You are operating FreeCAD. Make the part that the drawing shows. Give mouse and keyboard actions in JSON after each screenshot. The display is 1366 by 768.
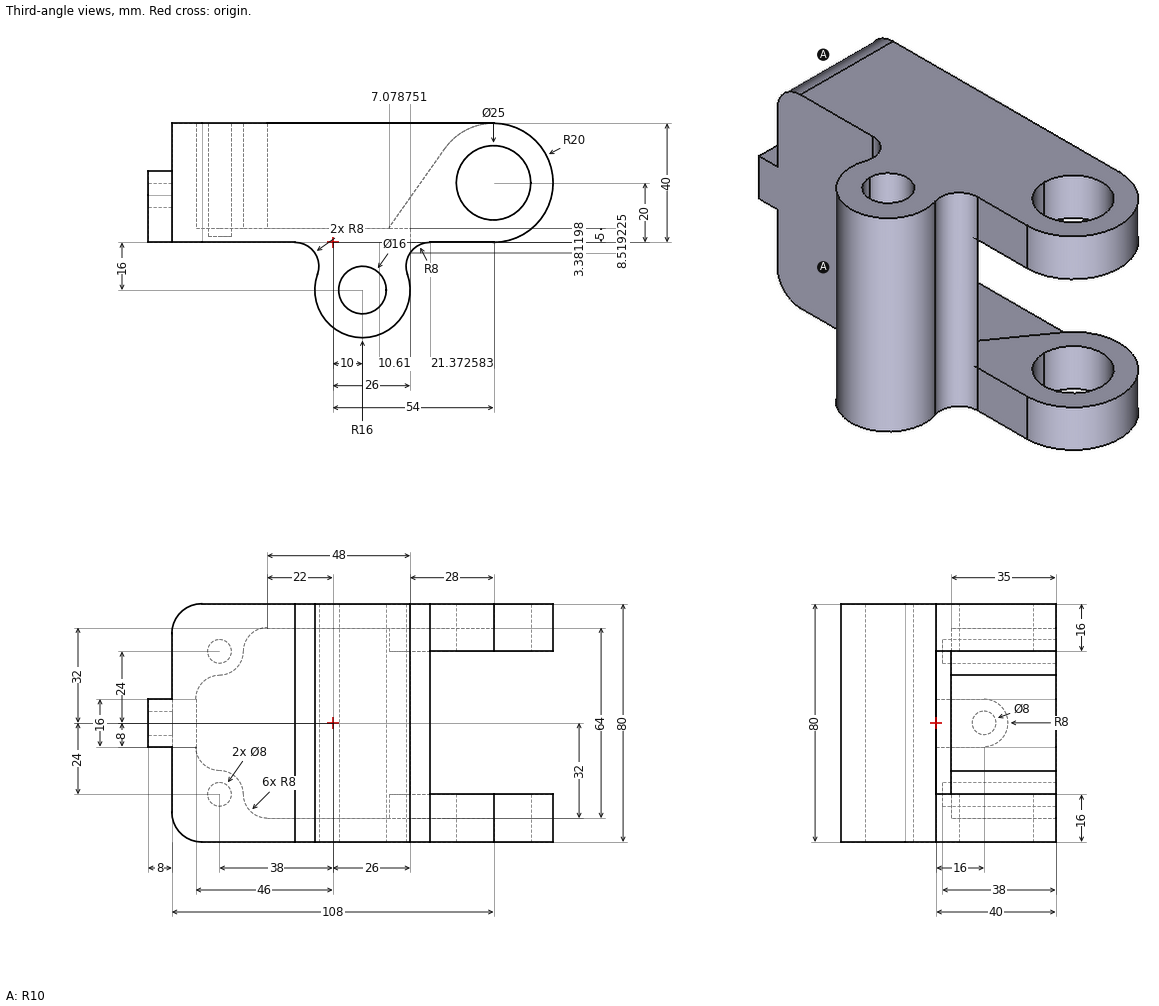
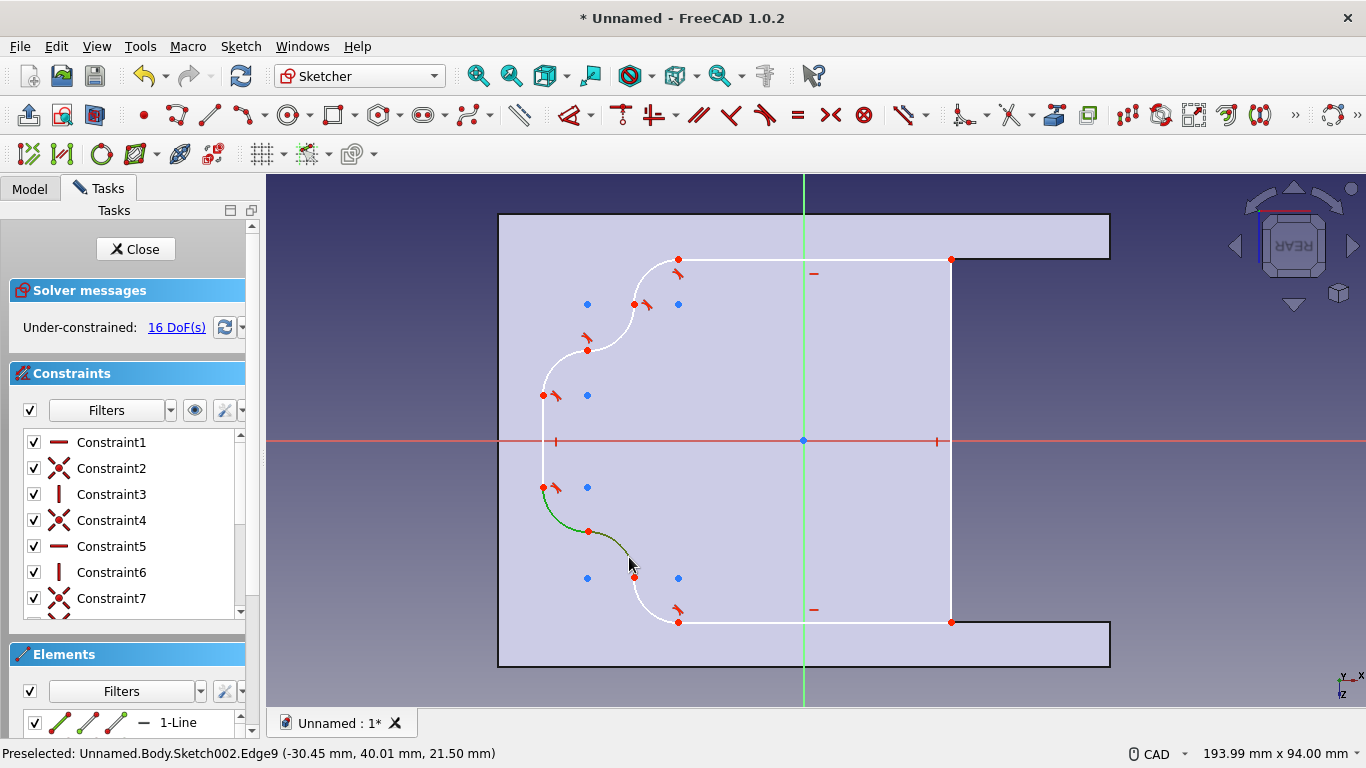
{"action": "key", "text": "t"}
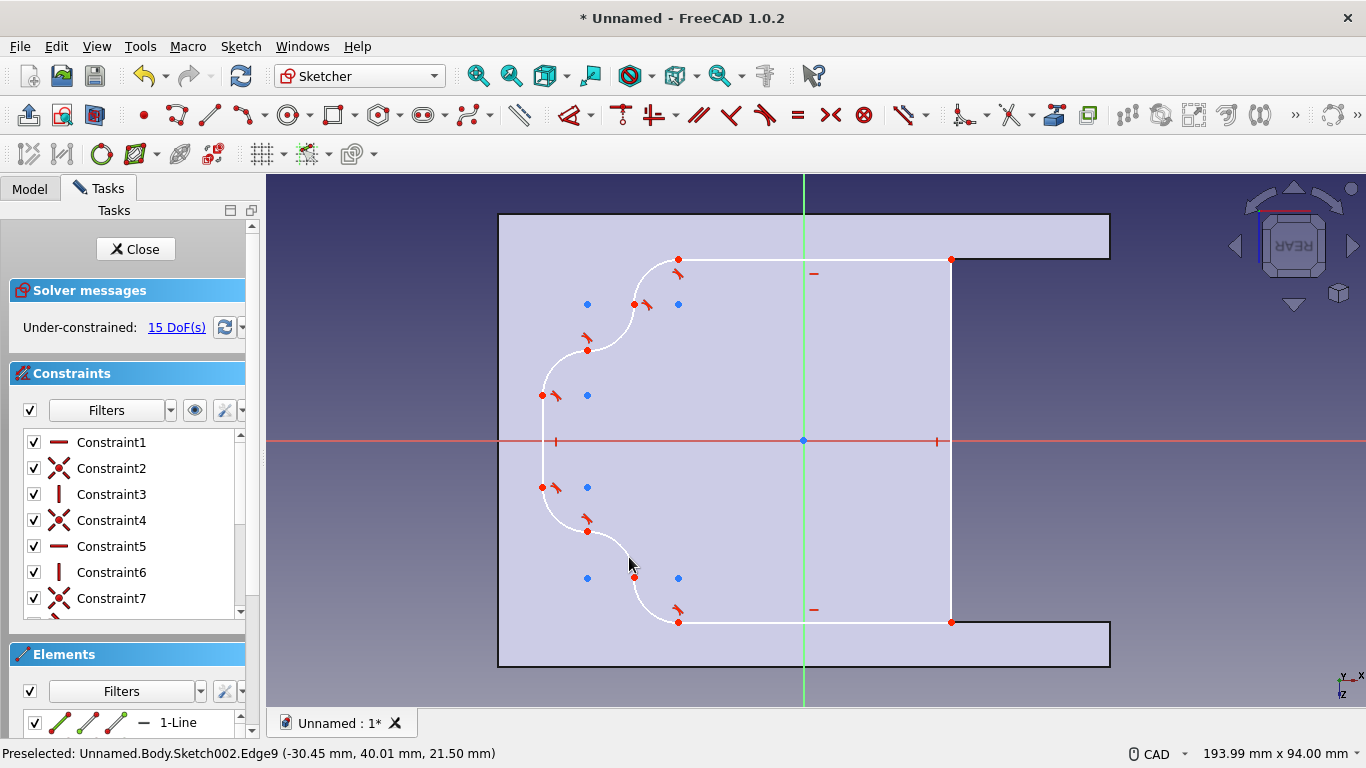
{"action": "left_click", "coordinate": [629, 557]}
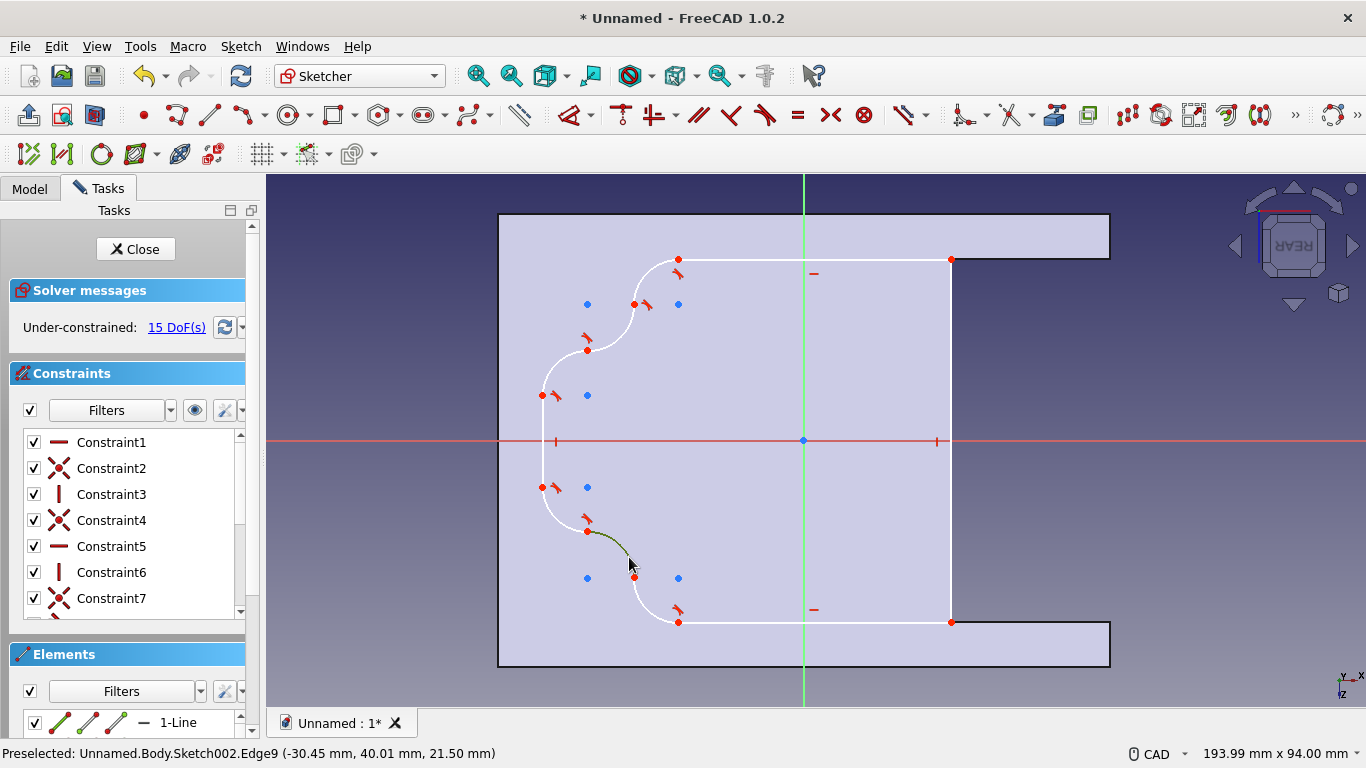
{"action": "left_click", "coordinate": [639, 598]}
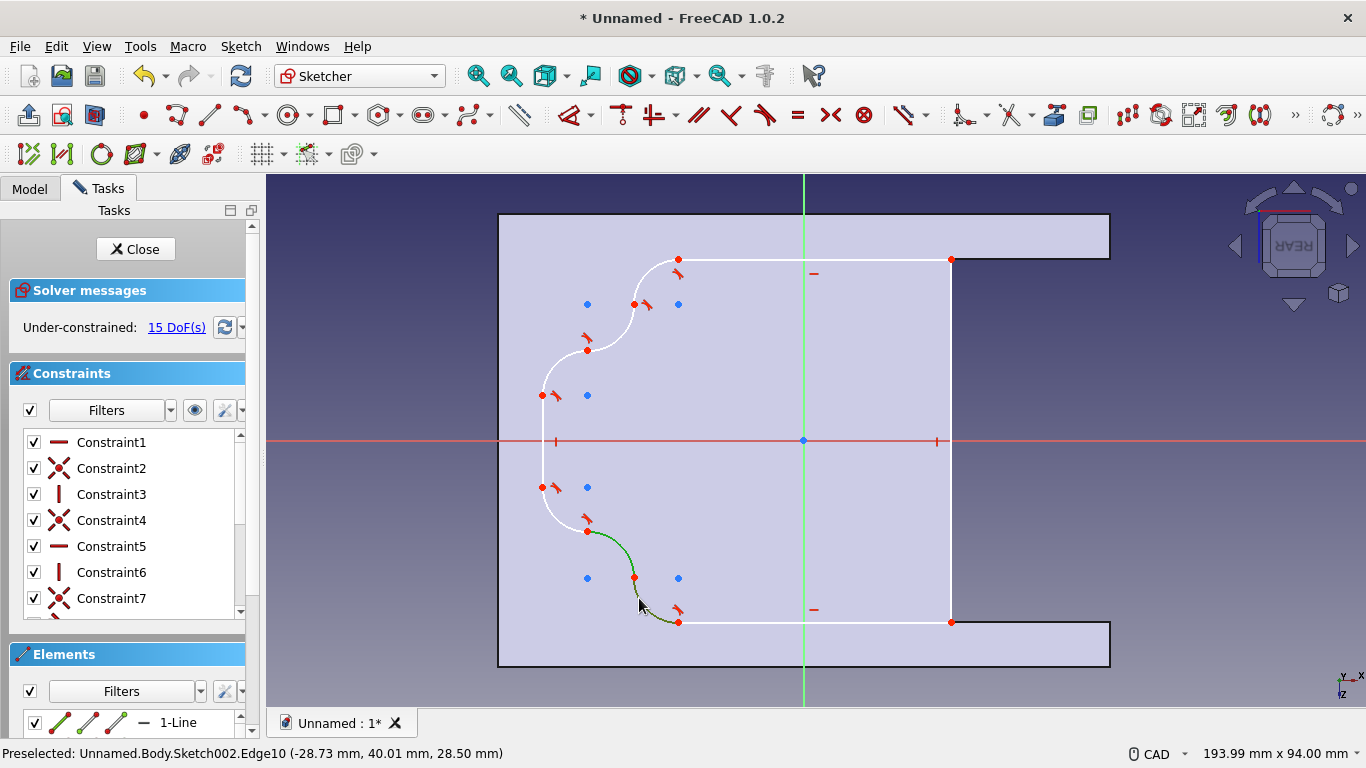
{"action": "key", "text": "t"}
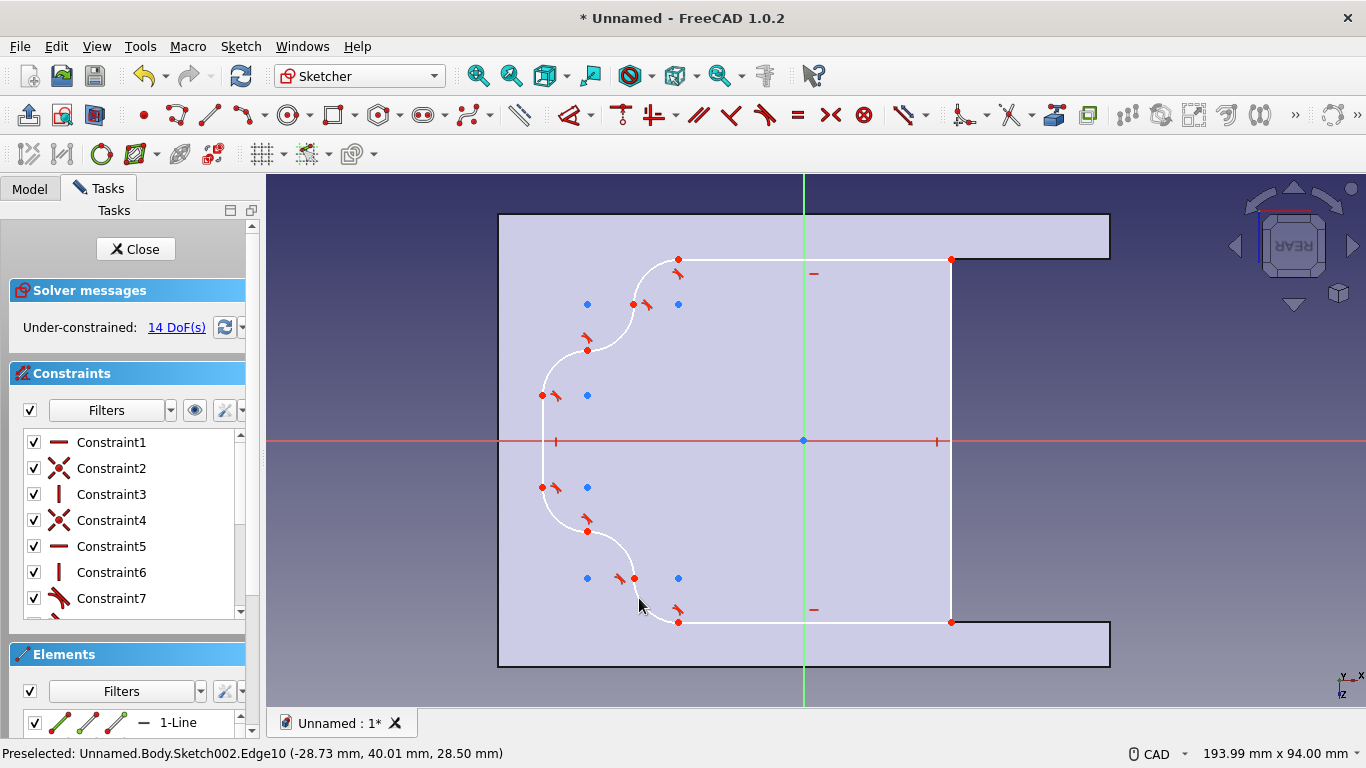
{"action": "left_click", "coordinate": [659, 265]}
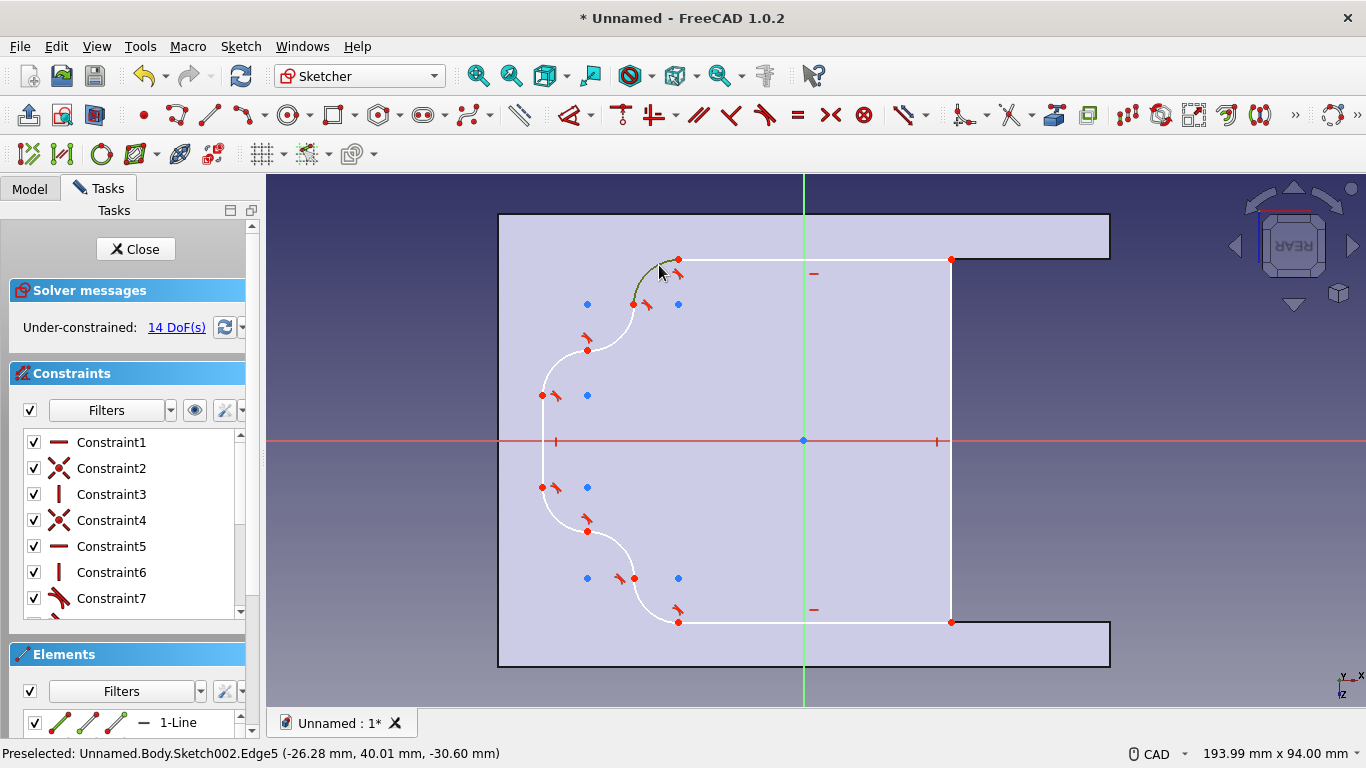
{"action": "left_click", "coordinate": [609, 346]}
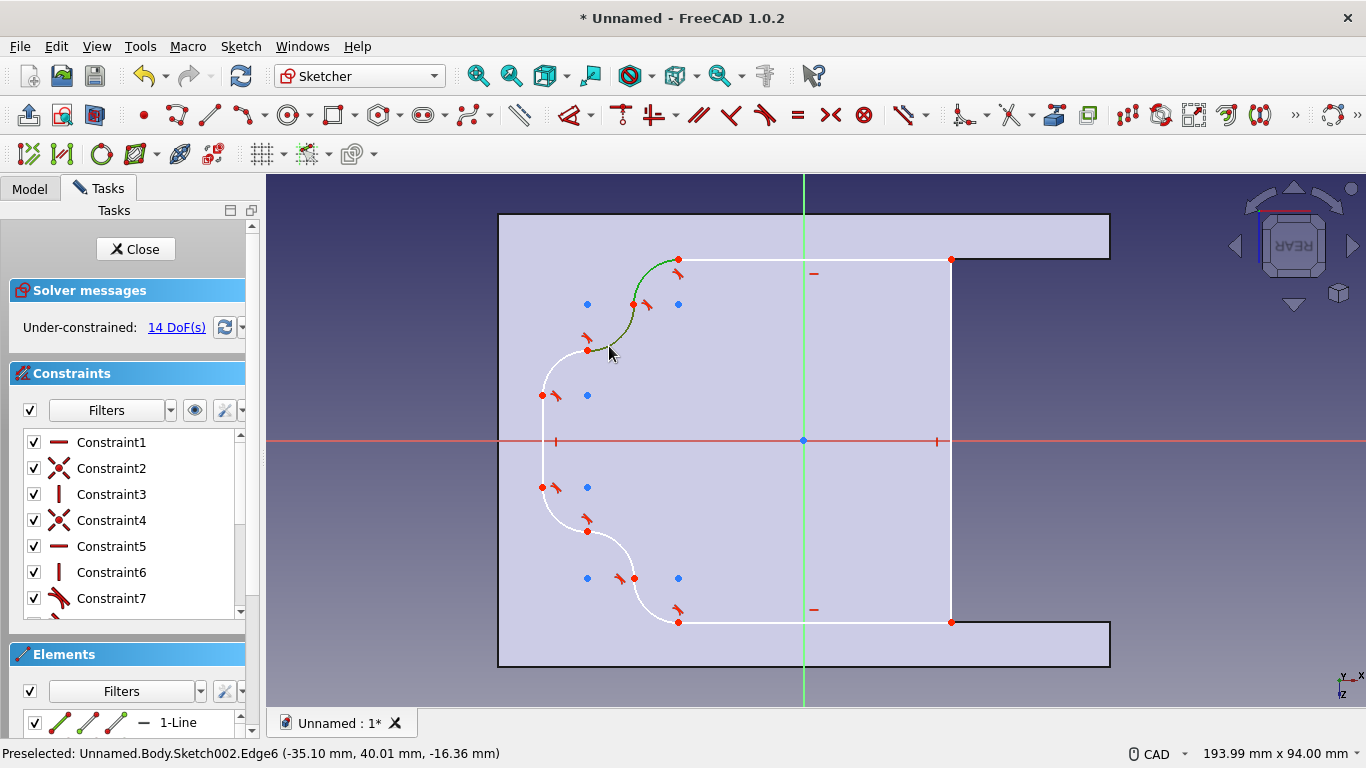
{"action": "left_click", "coordinate": [568, 356]}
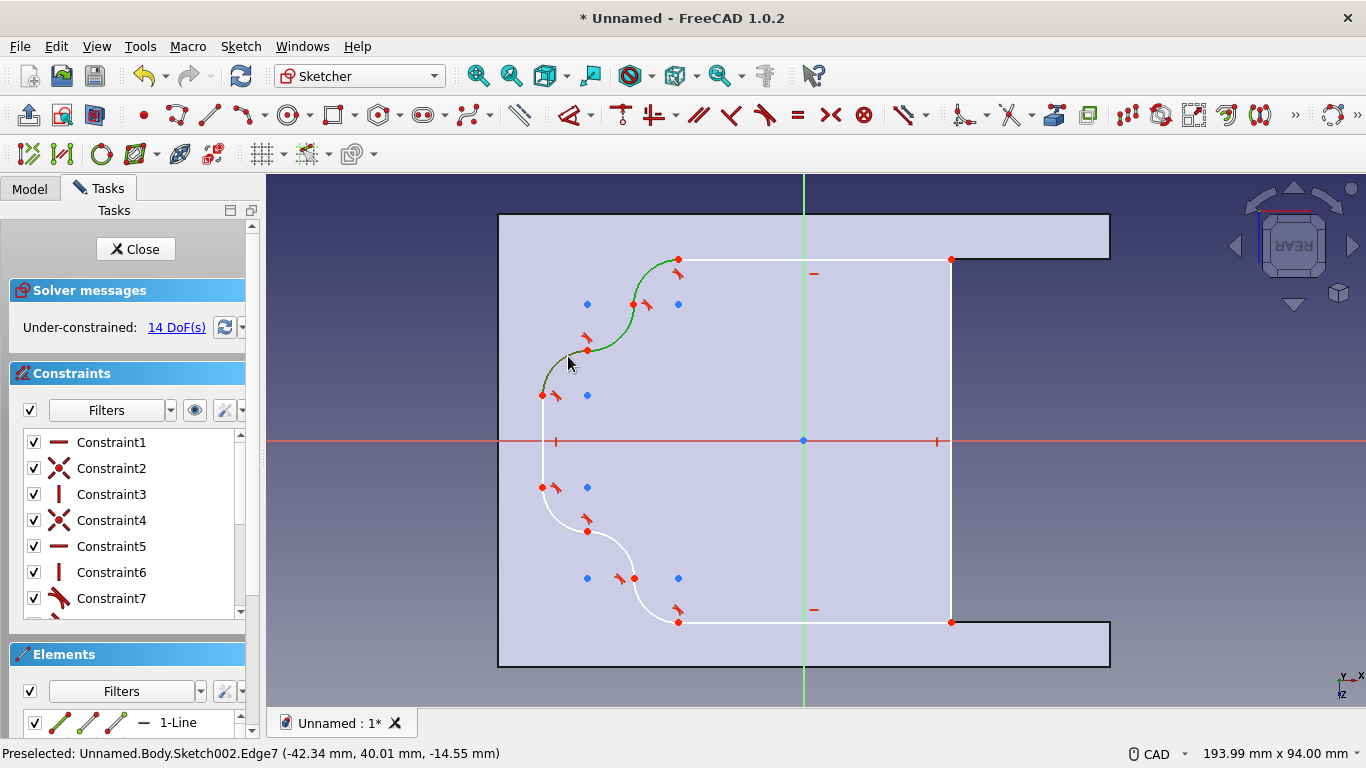
{"action": "left_click", "coordinate": [548, 507]}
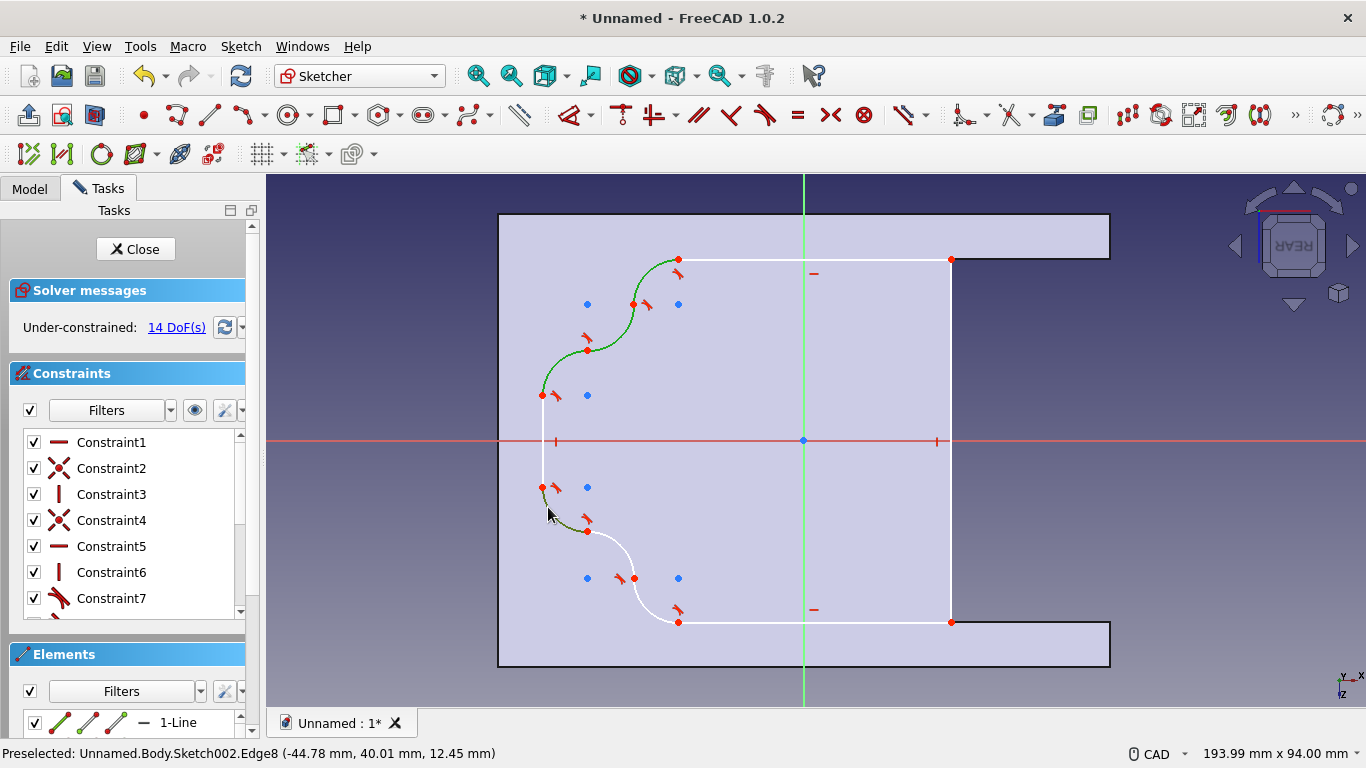
{"action": "left_click", "coordinate": [629, 557]}